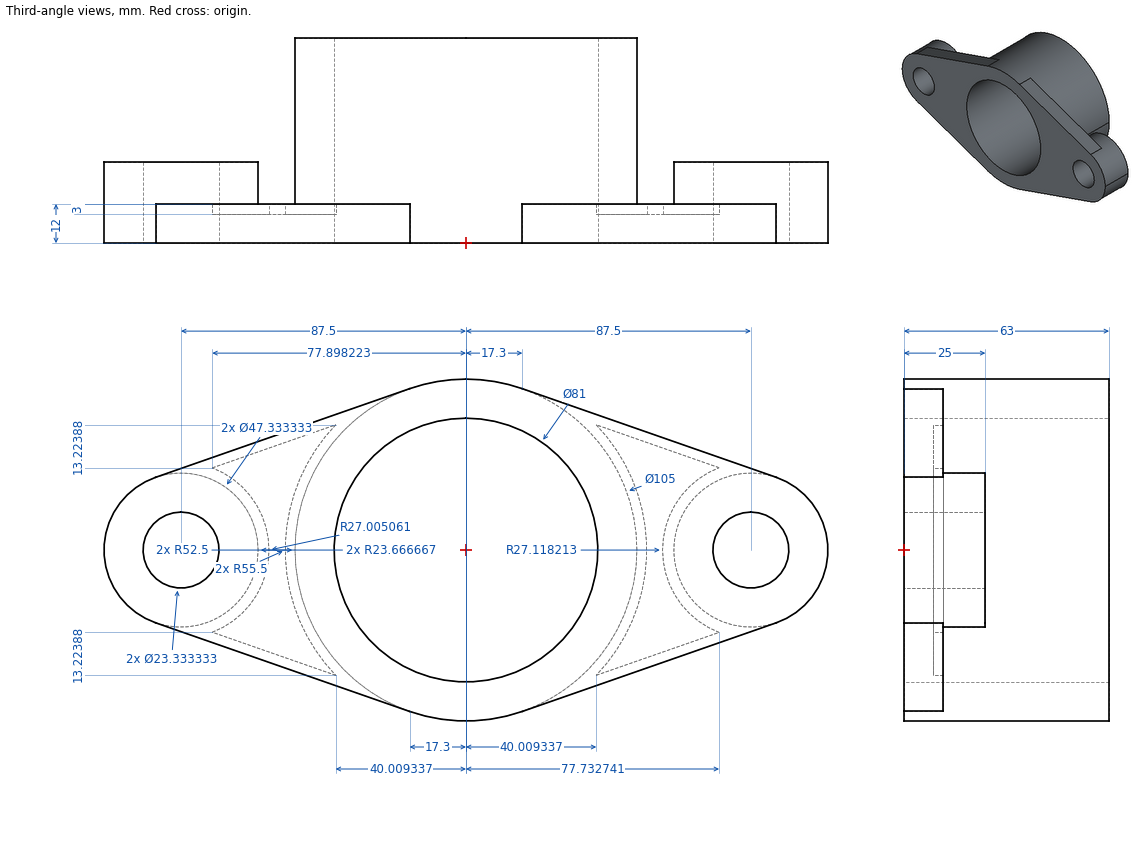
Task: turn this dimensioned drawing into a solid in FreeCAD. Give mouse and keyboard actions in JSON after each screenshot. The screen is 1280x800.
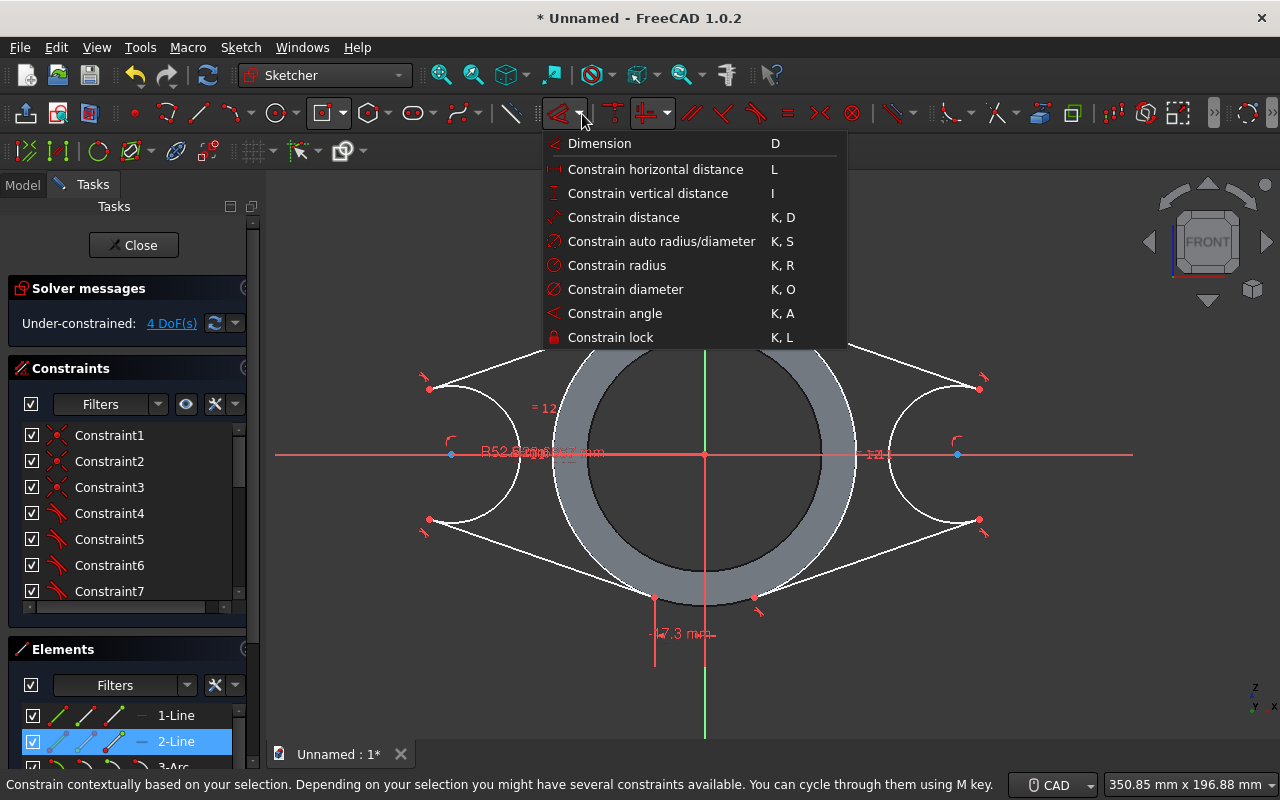
{"action": "left_click", "coordinate": [695, 169]}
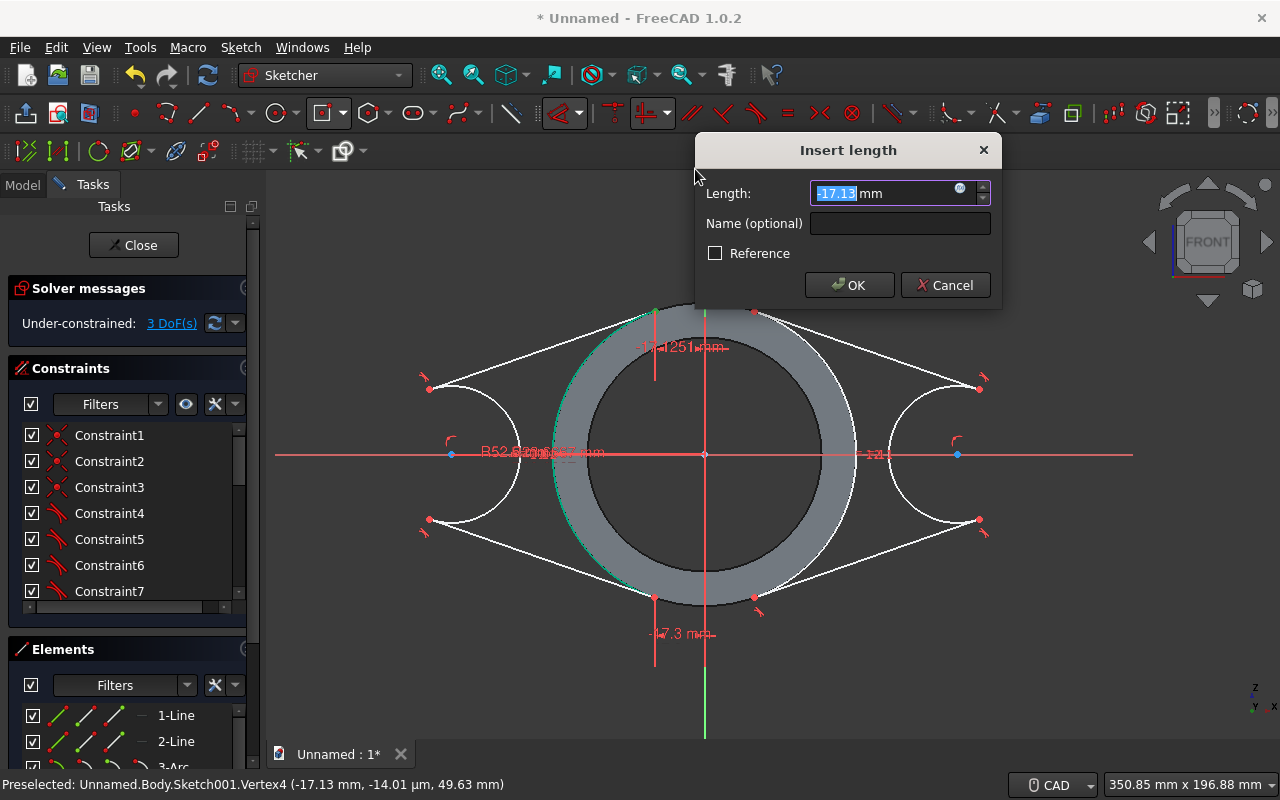
{"action": "type", "text": "-17.3"}
{"action": "key", "text": "Return"}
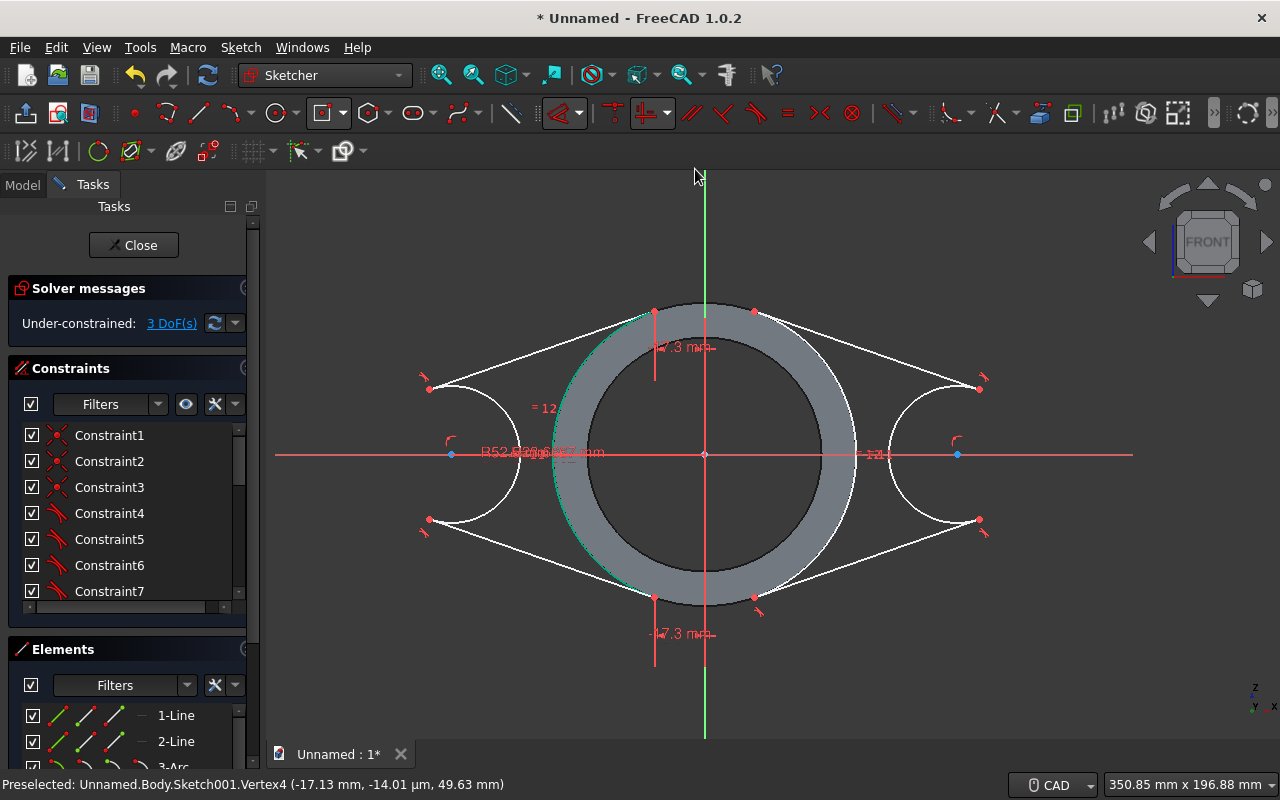
{"action": "left_click", "coordinate": [755, 311]}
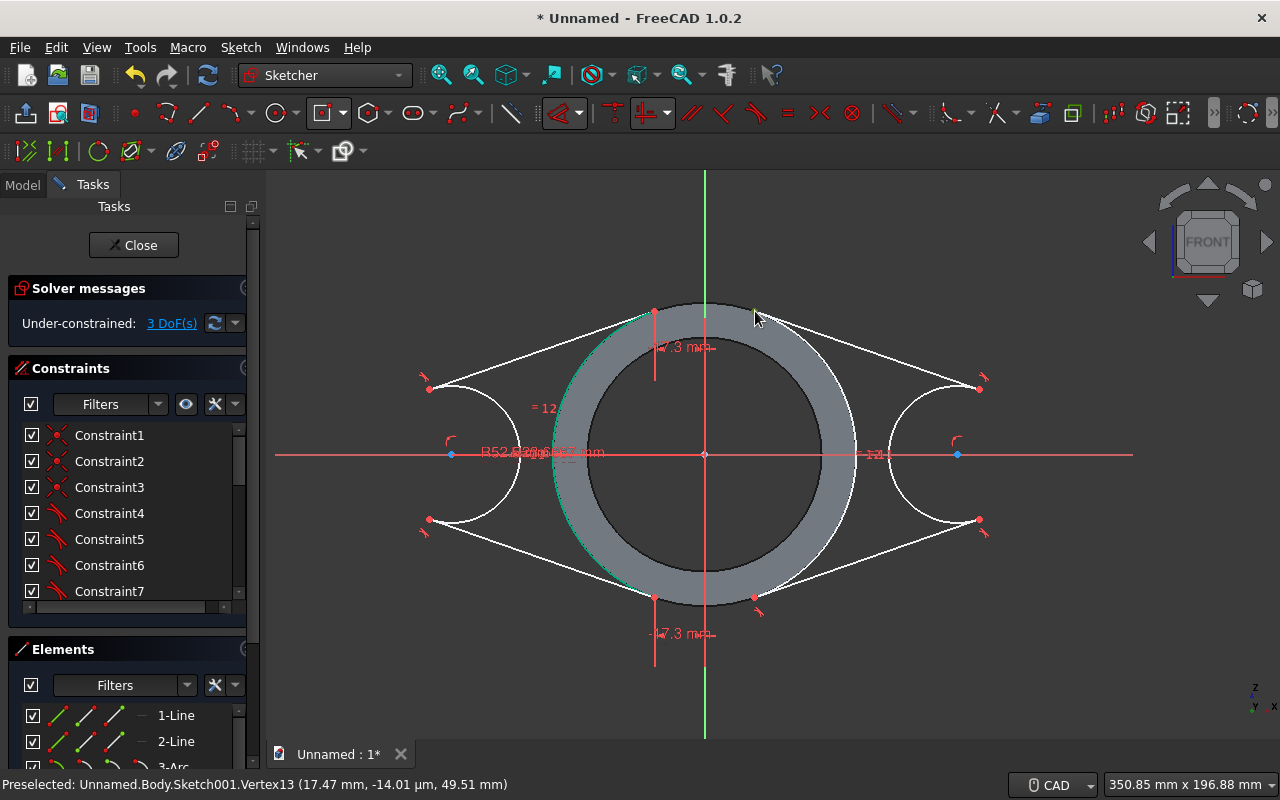
{"action": "key", "text": "l"}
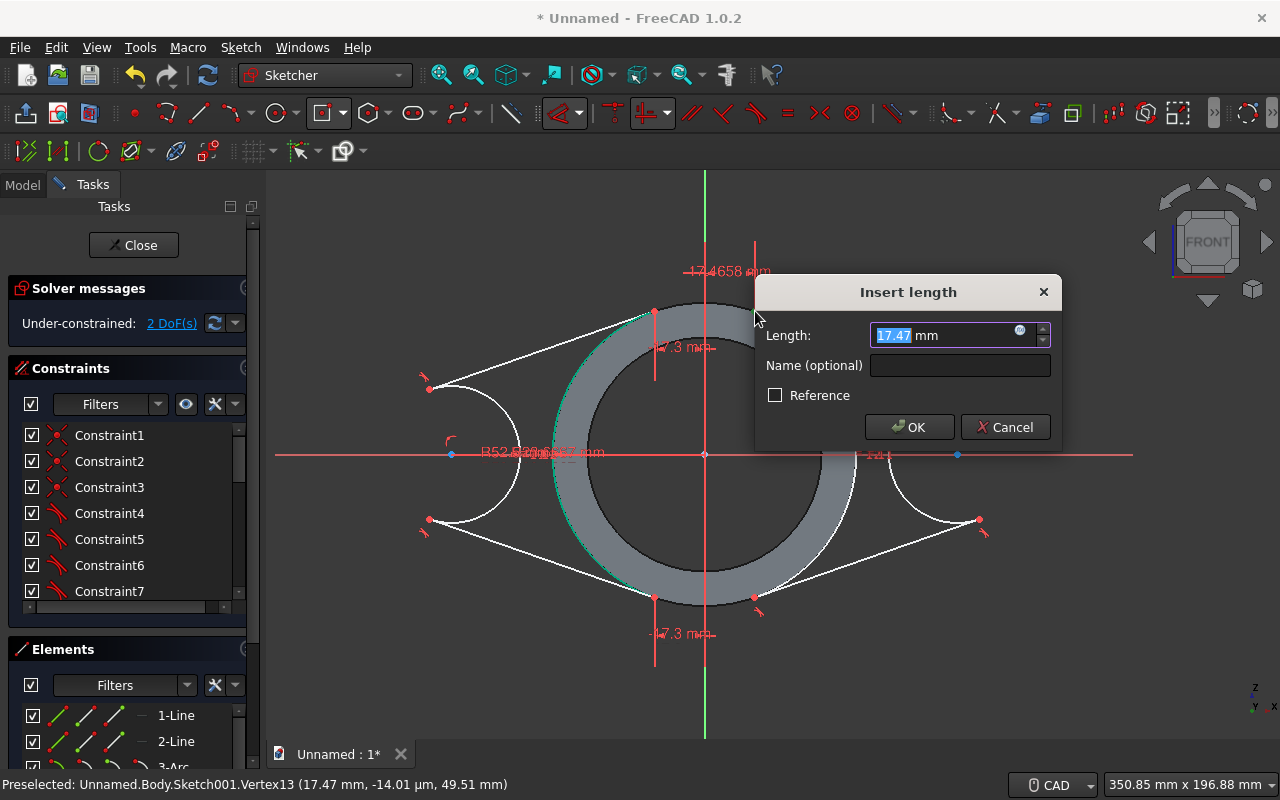
{"action": "type", "text": "17.3"}
{"action": "key", "text": "Return"}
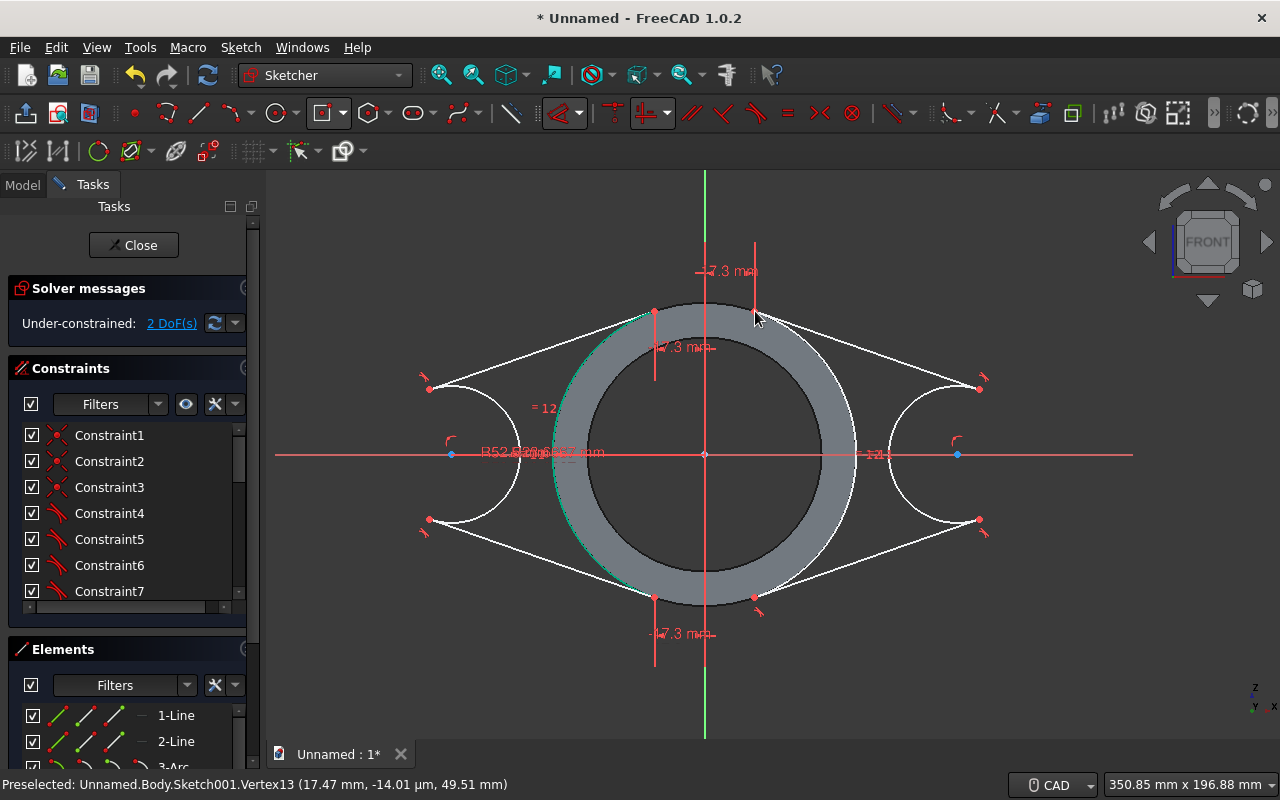
{"action": "left_click", "coordinate": [452, 455]}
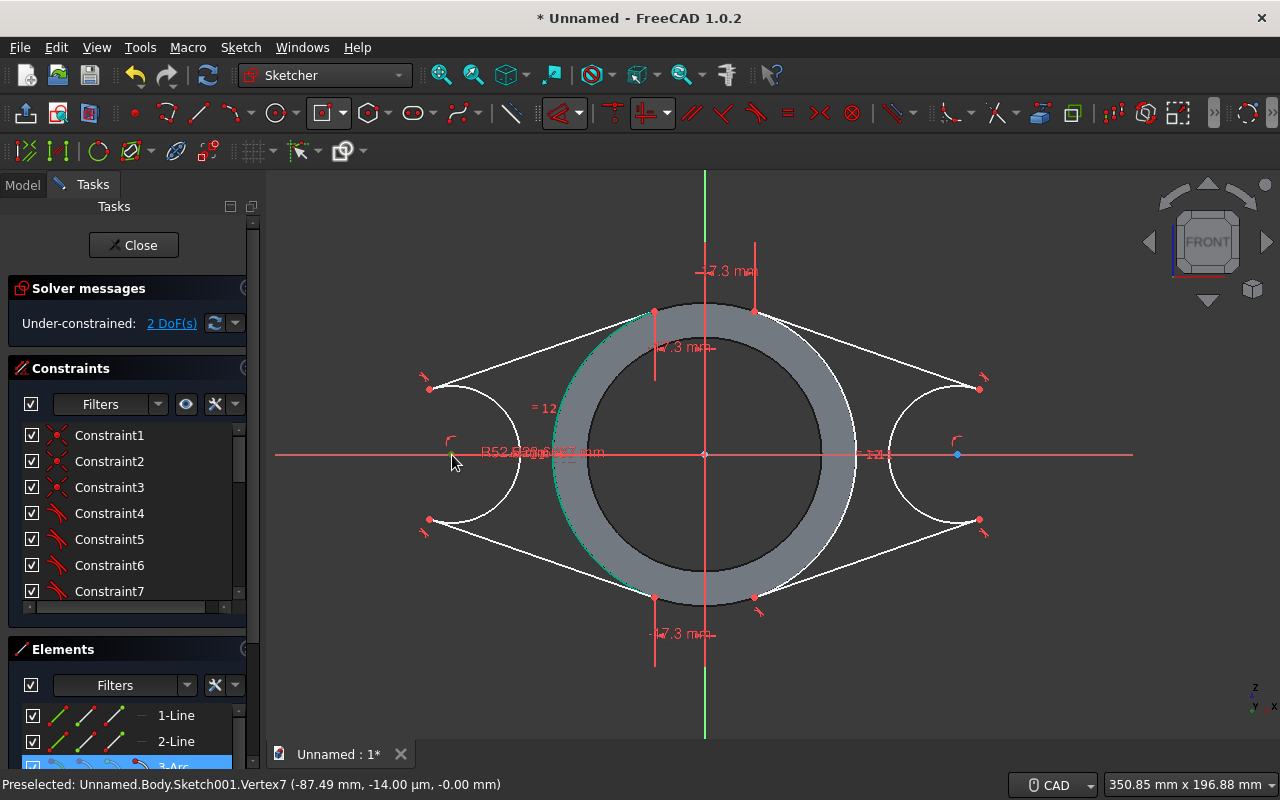
{"action": "key", "text": "l"}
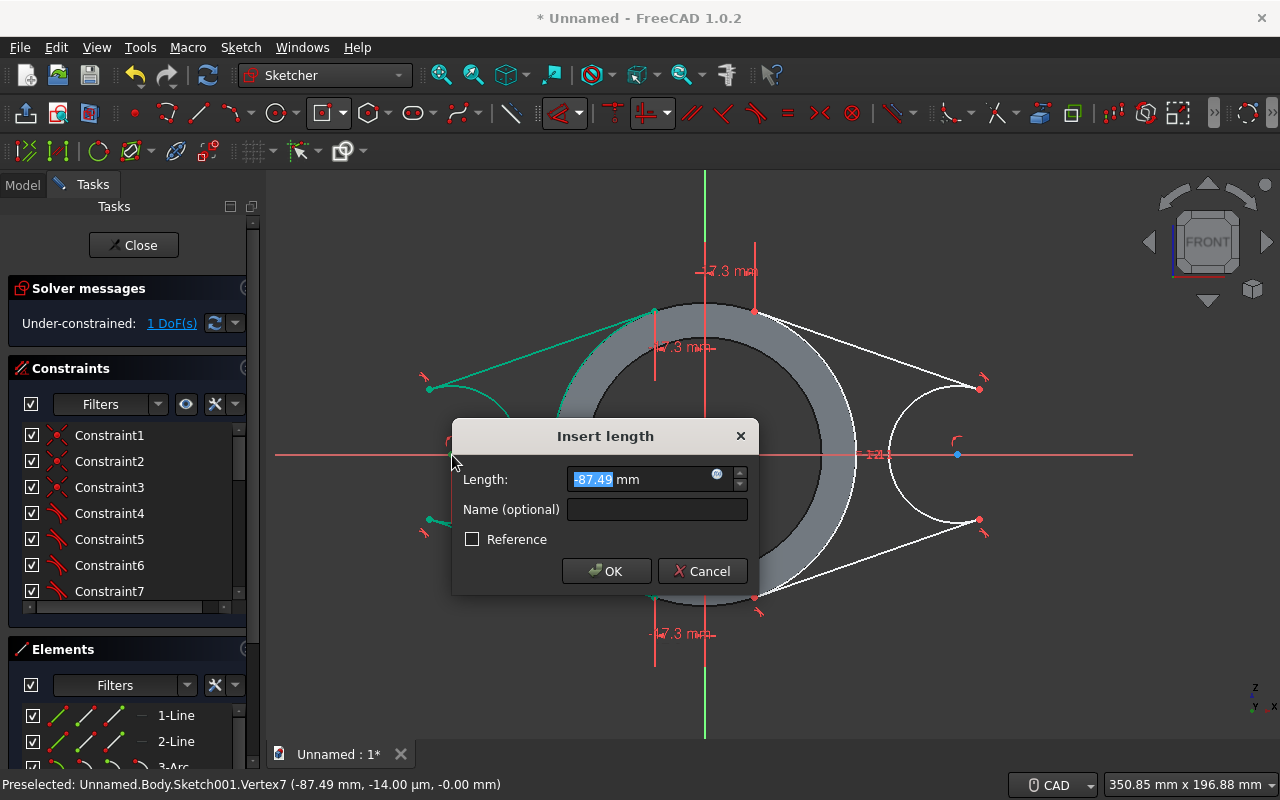
{"action": "type", "text": "-87.5"}
{"action": "key", "text": "Return"}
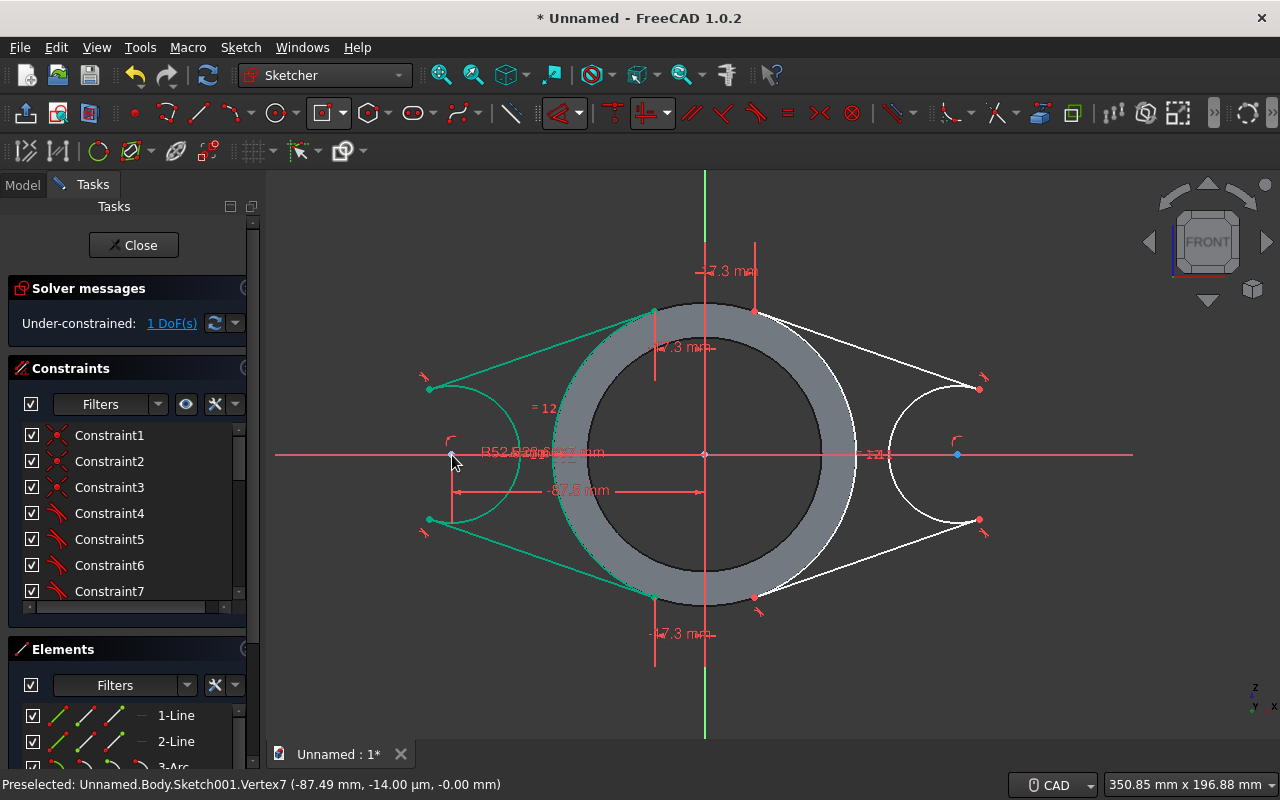
{"action": "left_click", "coordinate": [957, 455]}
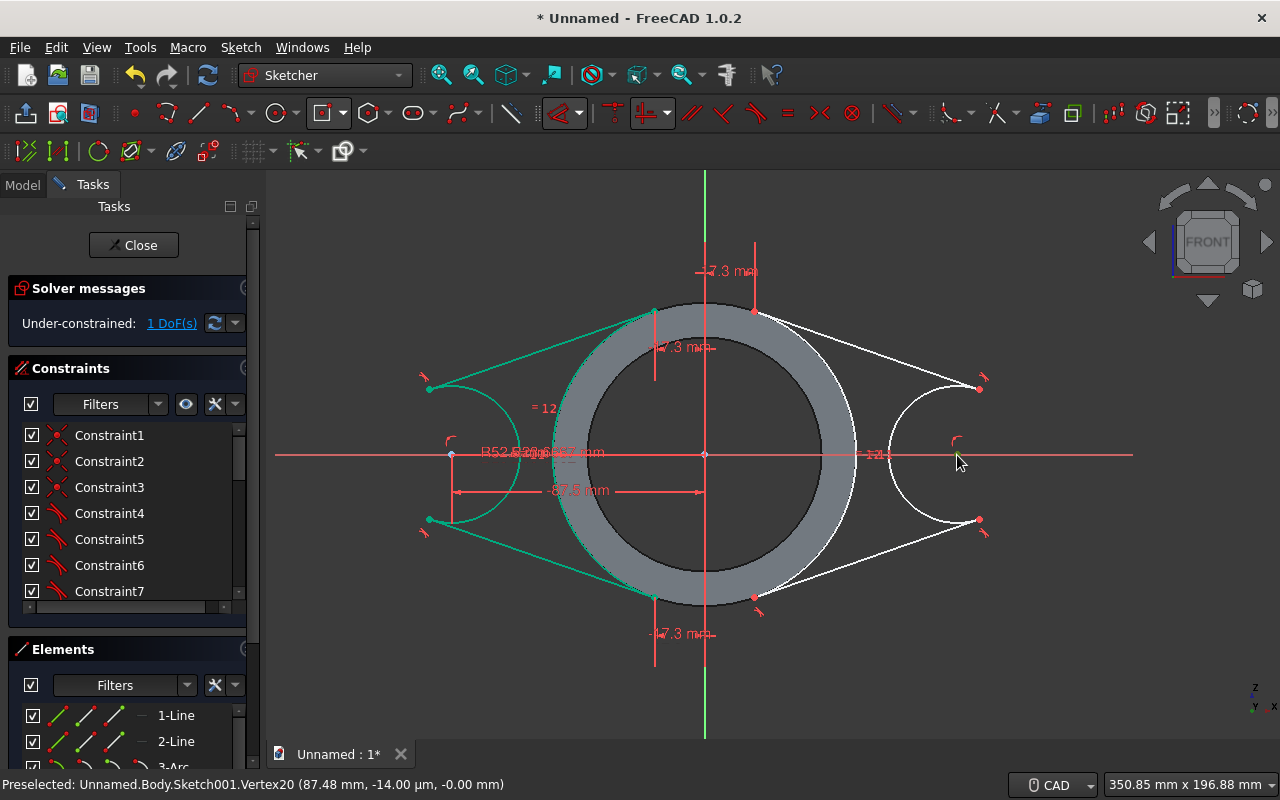
{"action": "key", "text": "l"}